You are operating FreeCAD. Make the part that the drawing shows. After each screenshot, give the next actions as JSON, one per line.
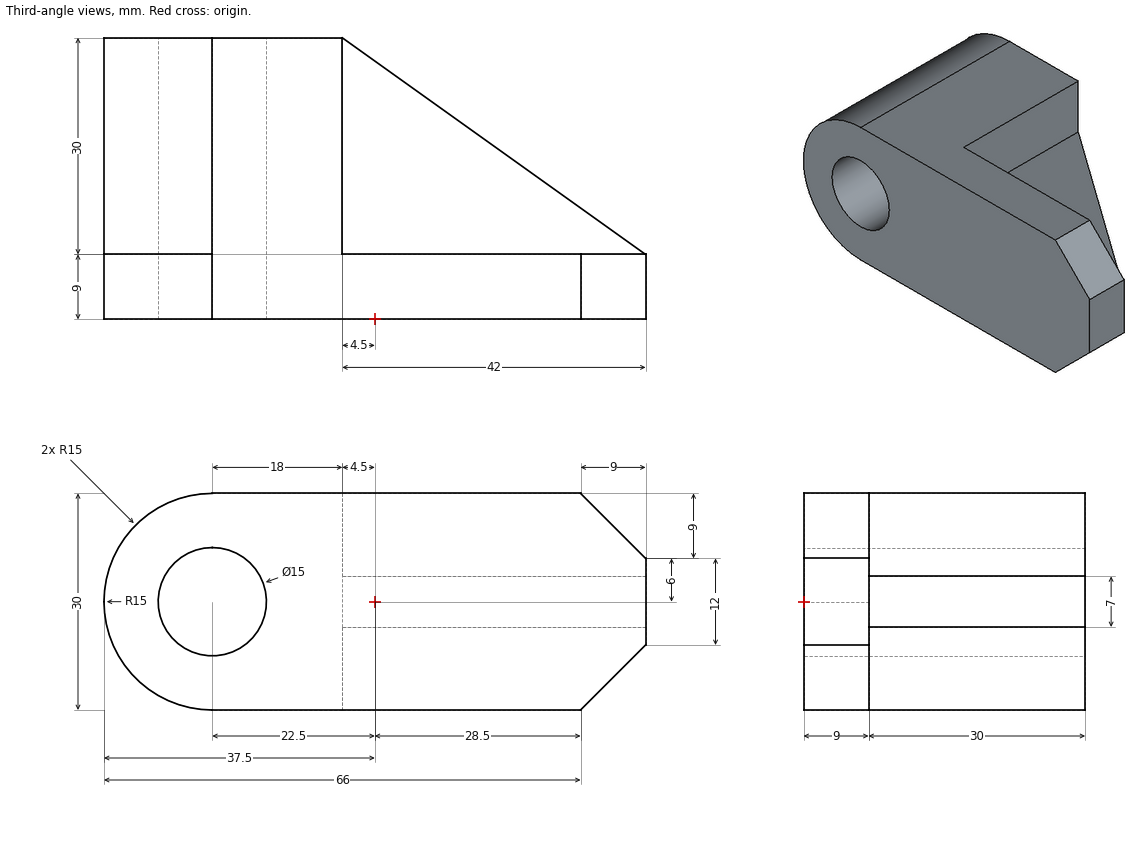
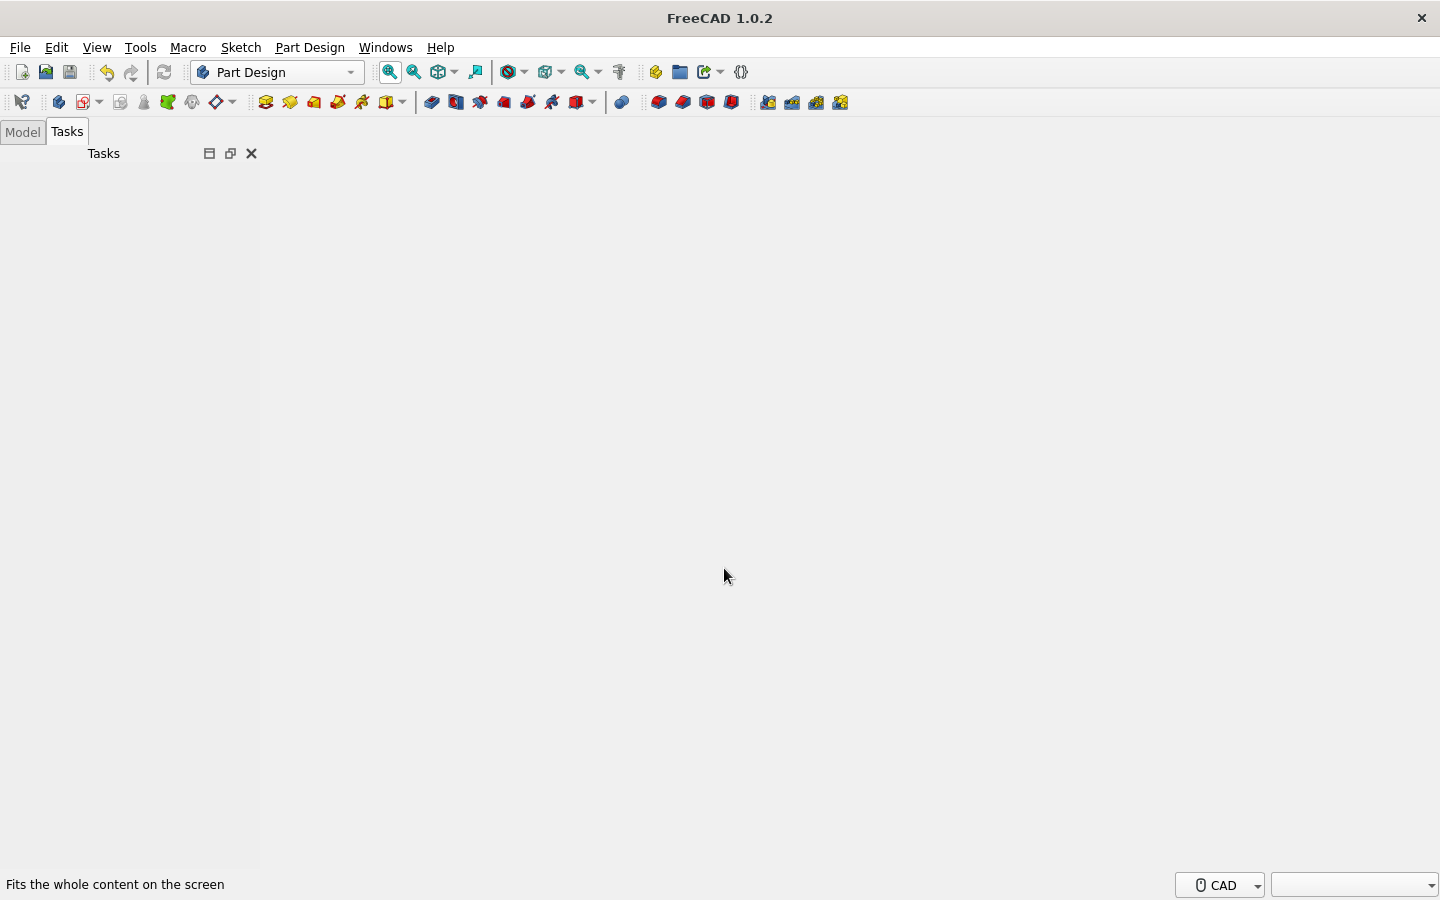
{"action": "key", "text": "ctrl+n"}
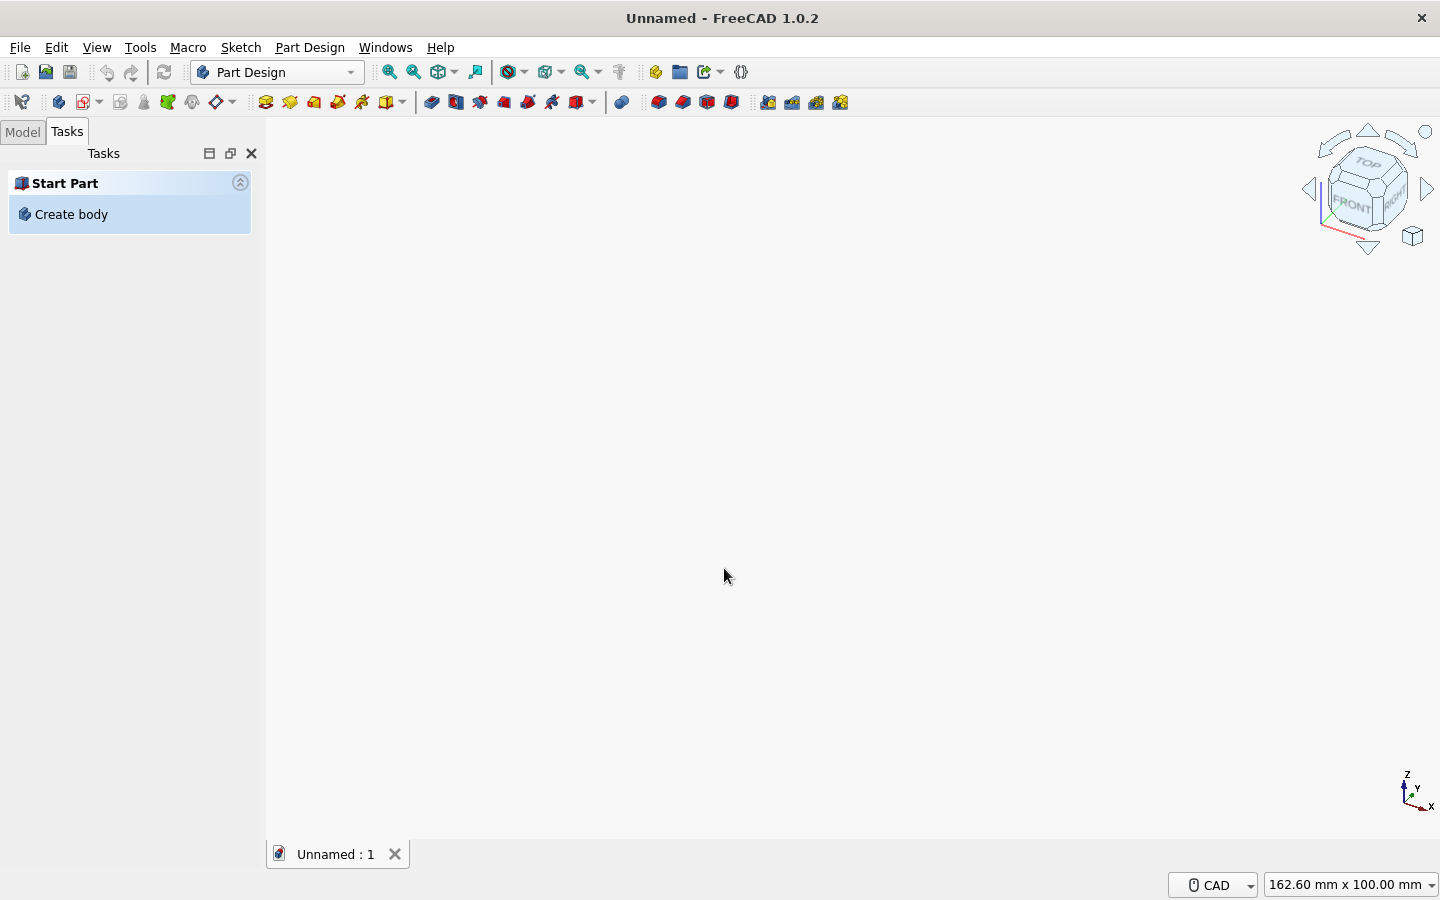
{"action": "left_click", "coordinate": [84, 102]}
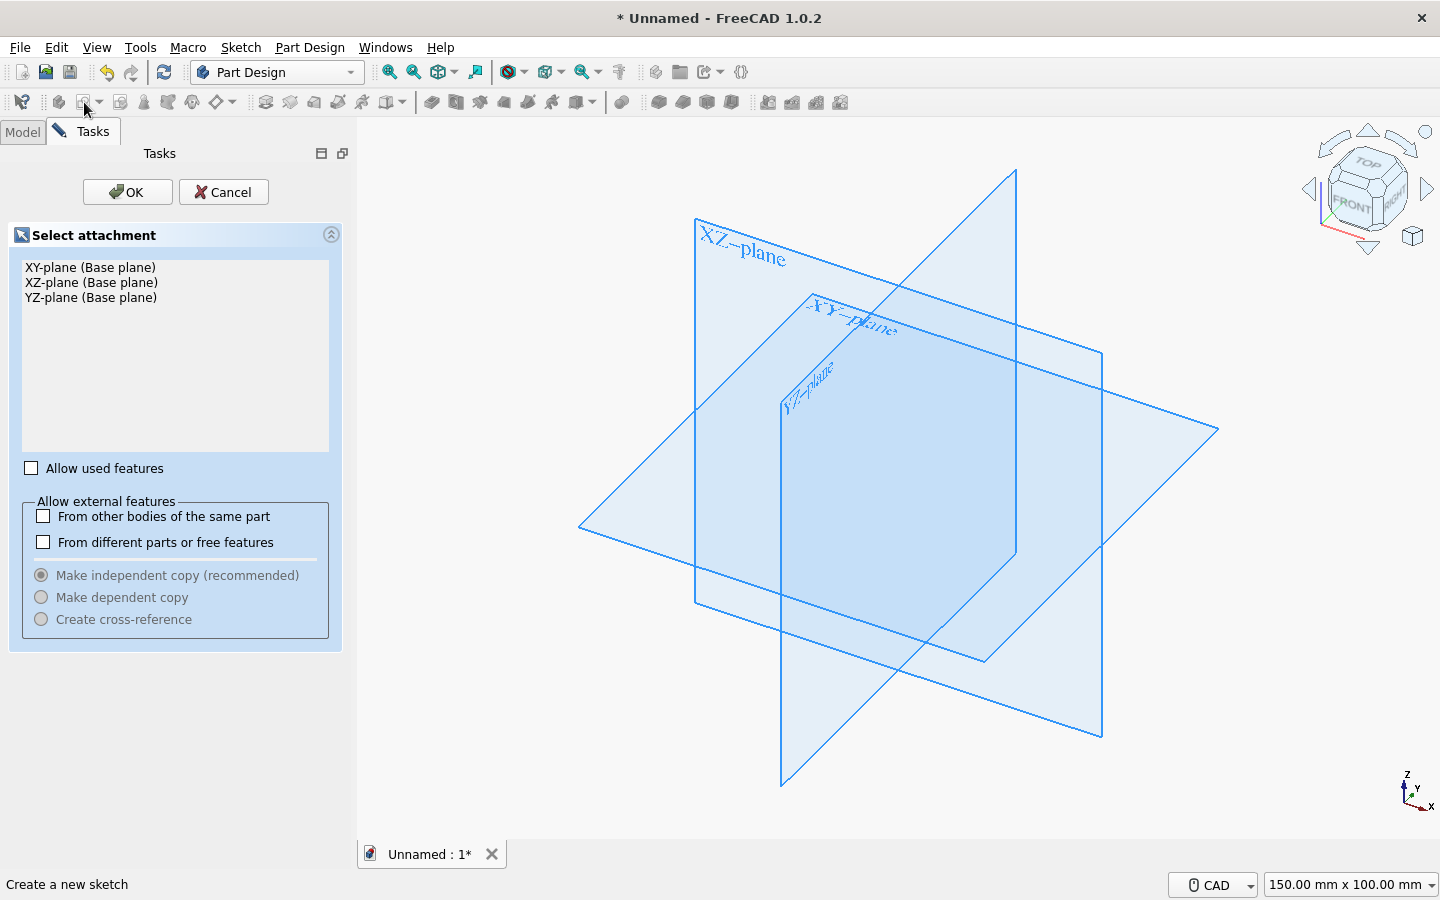
{"action": "left_click", "coordinate": [82, 282]}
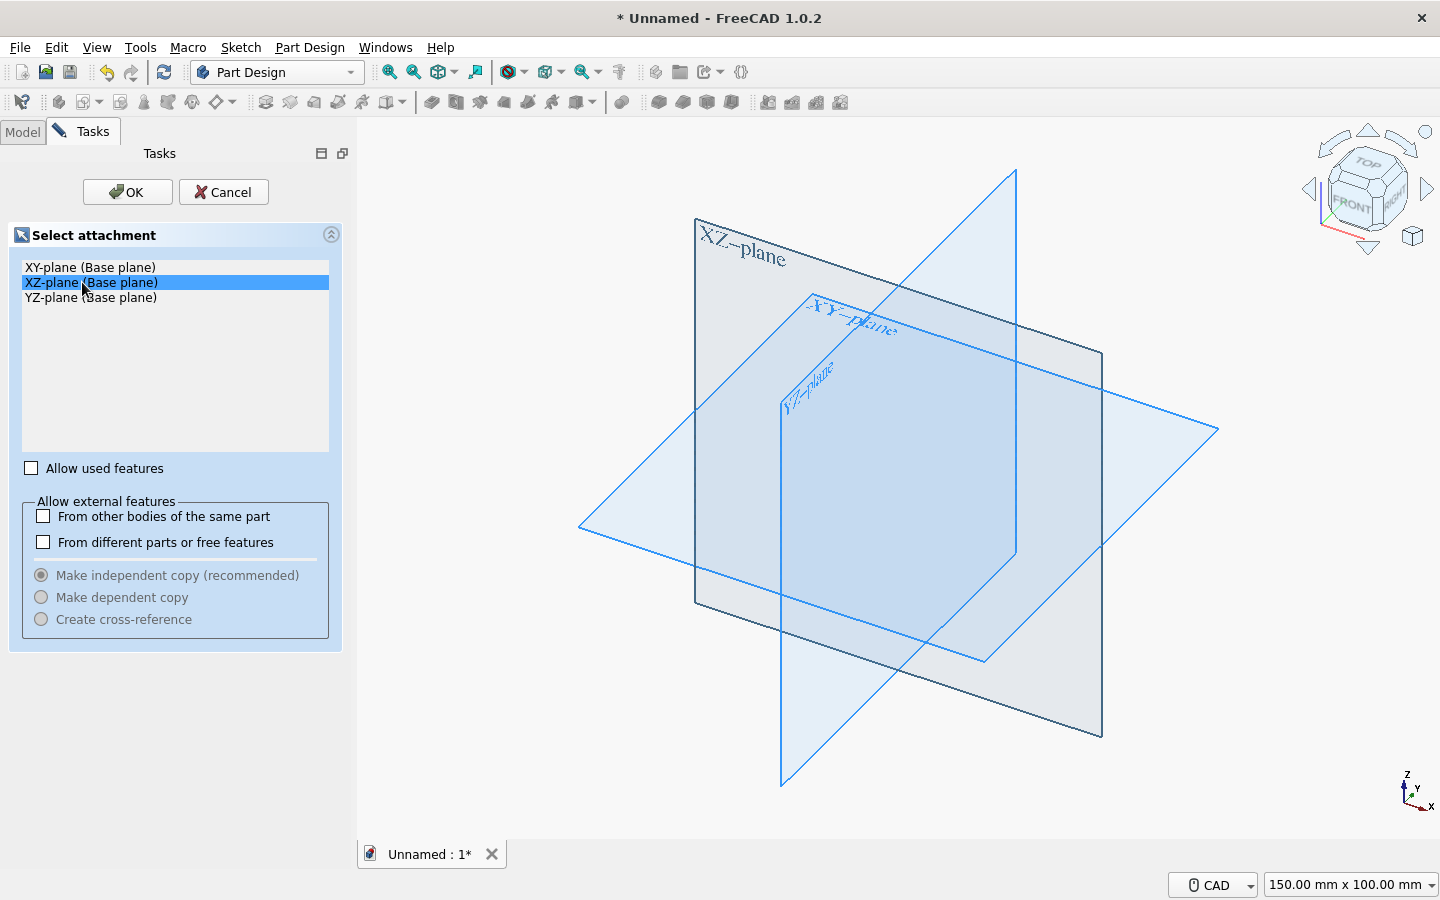
{"action": "left_click", "coordinate": [128, 192]}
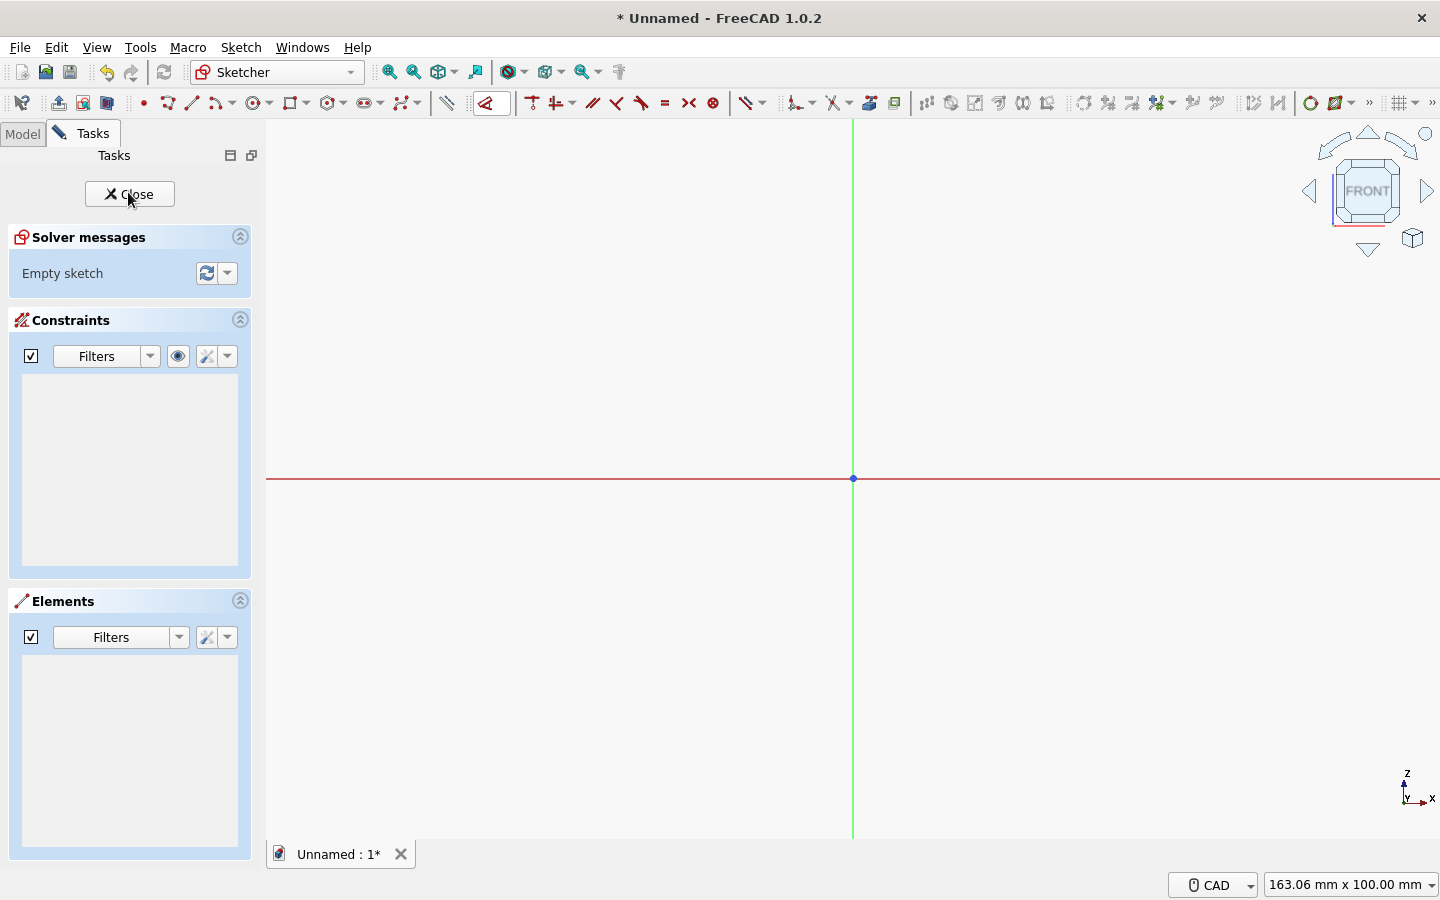
{"action": "key", "text": "g m"}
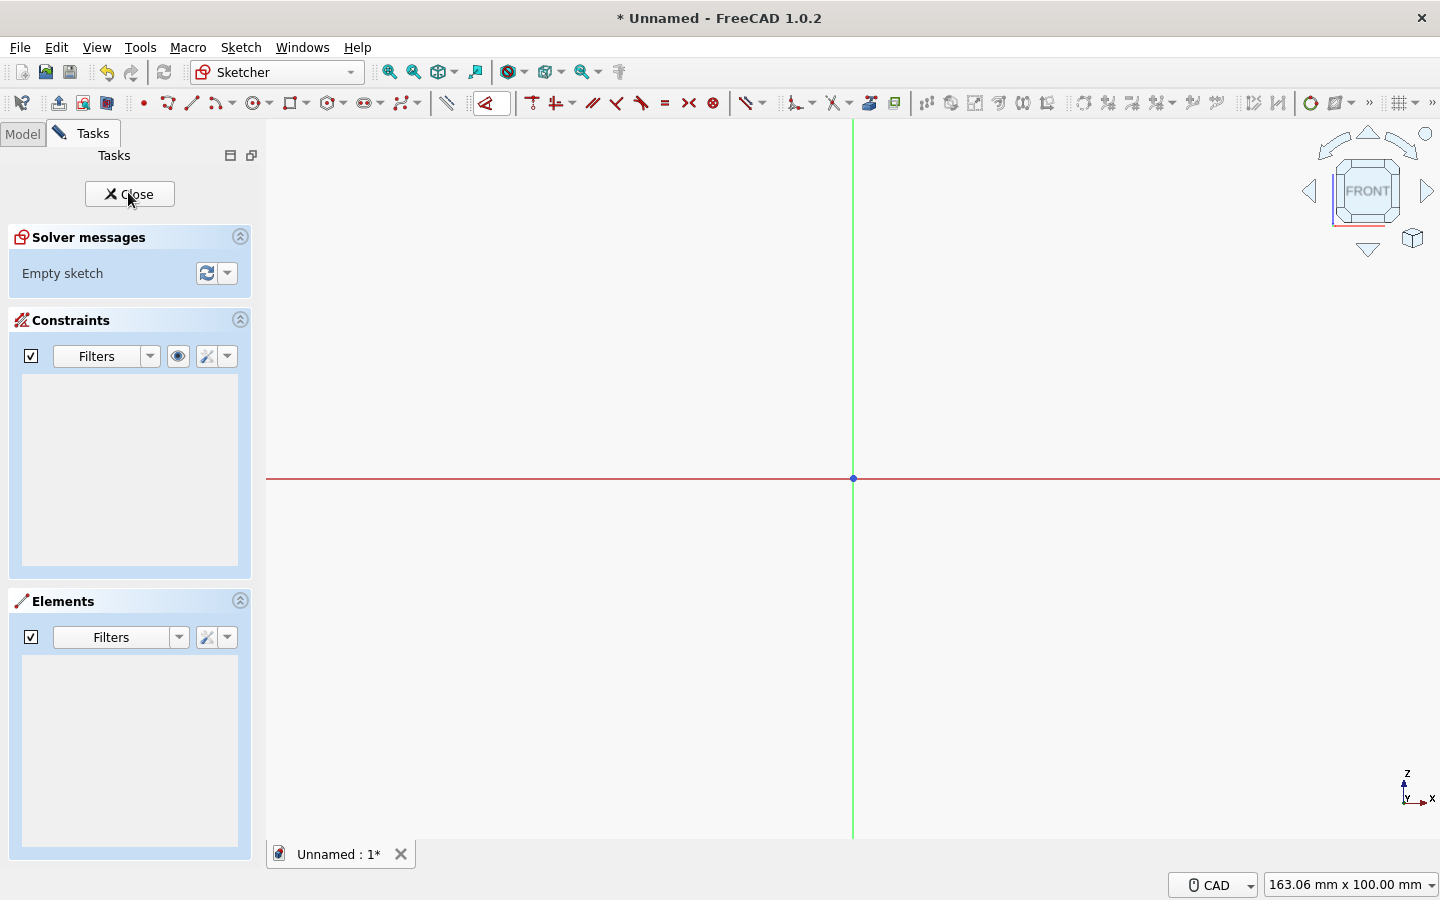
{"action": "left_click", "coordinate": [1058, 587]}
{"action": "left_click", "coordinate": [583, 587]}
{"action": "left_click", "coordinate": [583, 371]}
{"action": "left_click", "coordinate": [1058, 371]}
{"action": "left_click", "coordinate": [1123, 436]}
{"action": "left_click", "coordinate": [1123, 522]}
{"action": "left_click", "coordinate": [1058, 588]}
{"action": "key", "text": "Escape"}
{"action": "key", "text": "Escape"}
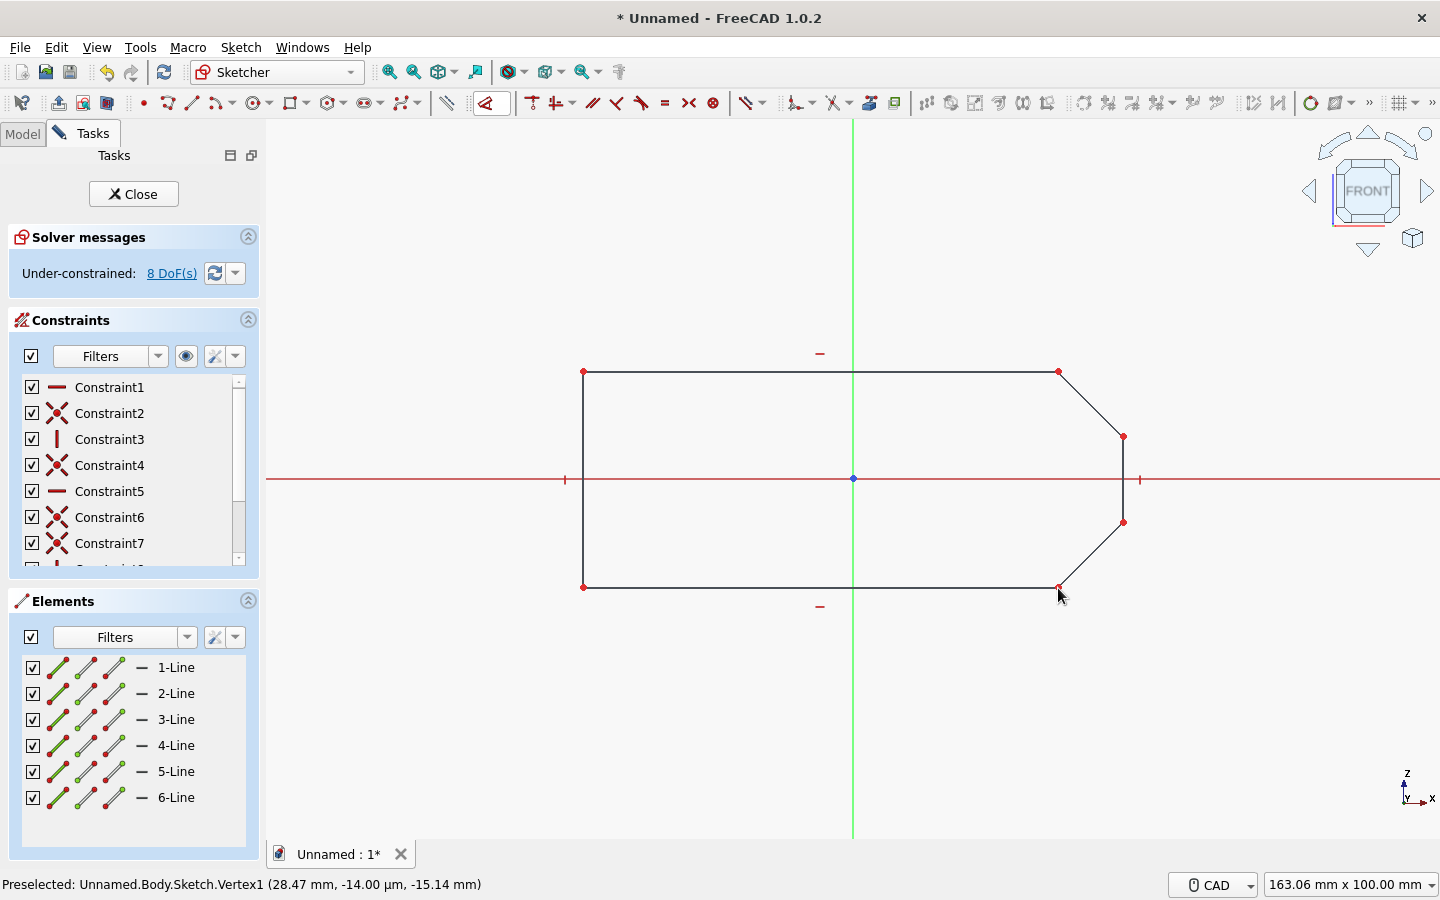
{"action": "key", "text": "d"}